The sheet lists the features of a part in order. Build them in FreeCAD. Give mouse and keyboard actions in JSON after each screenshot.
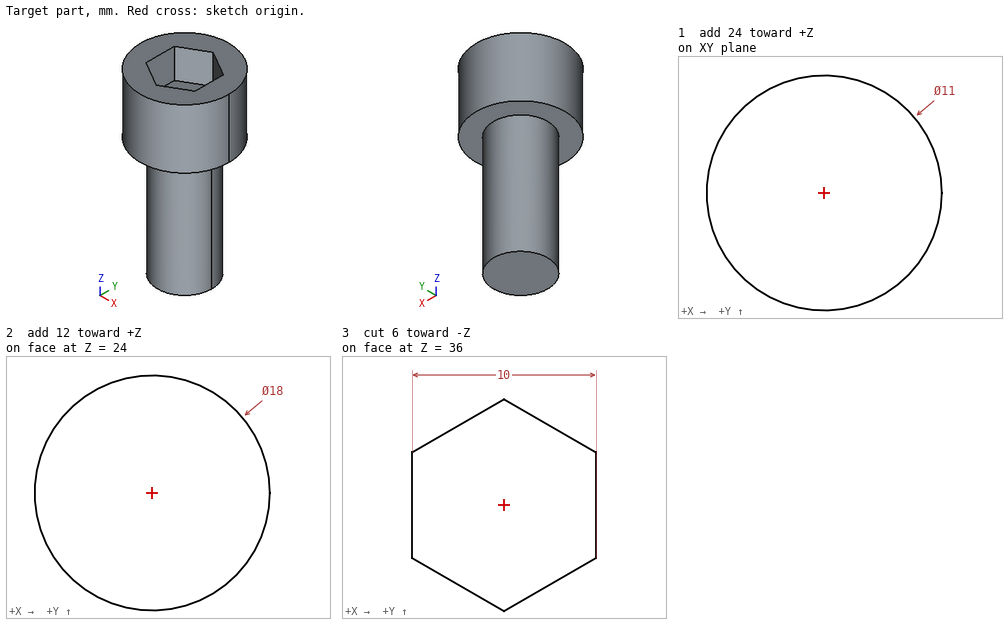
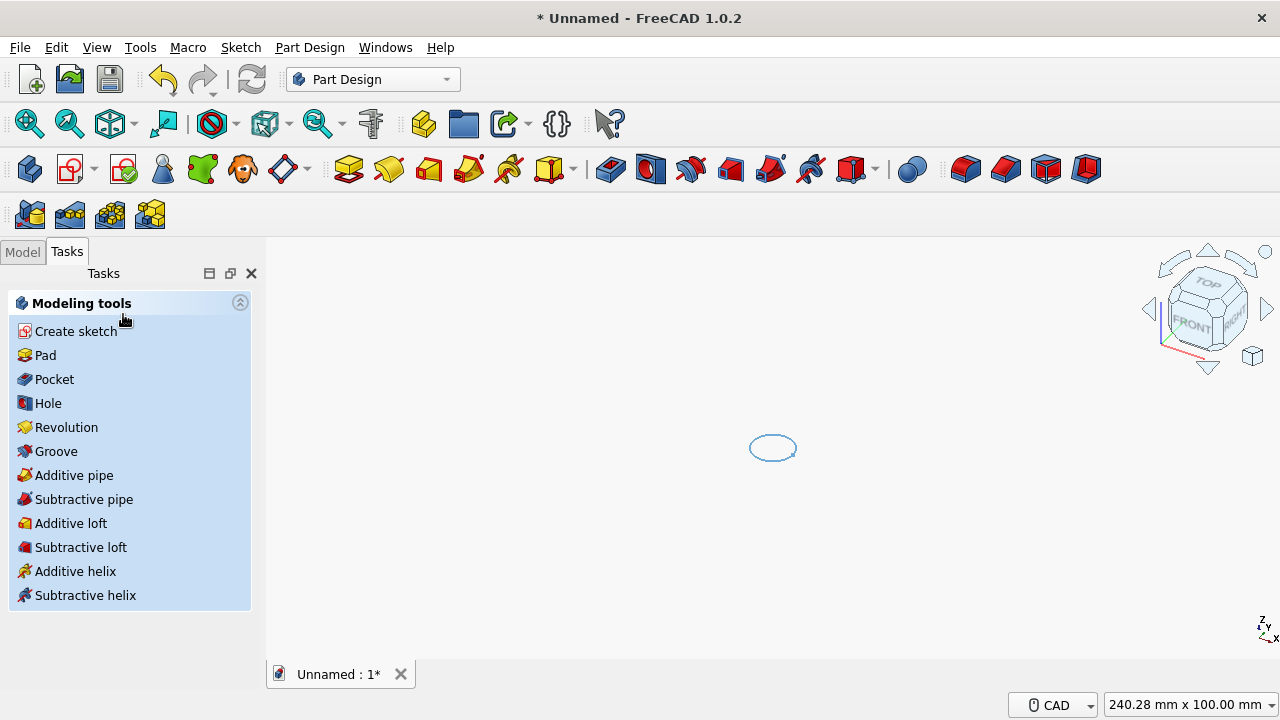
{"action": "left_click", "coordinate": [350, 170]}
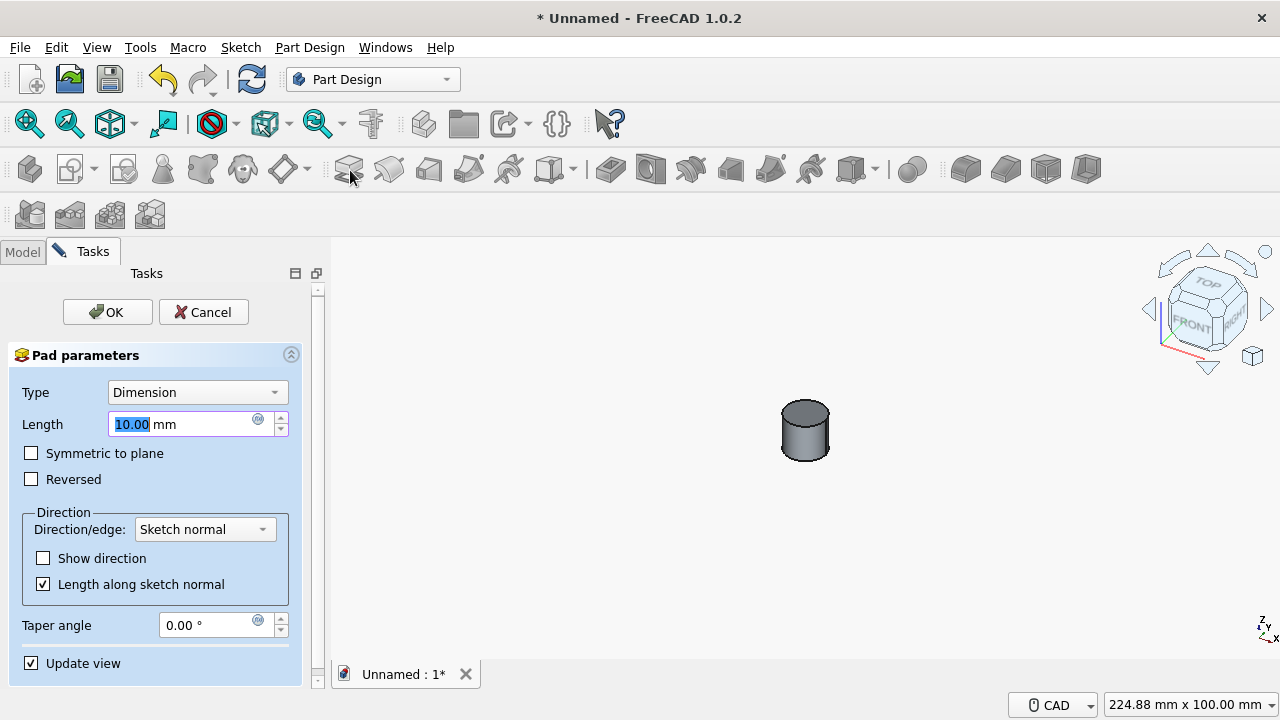
{"action": "type", "text": "24"}
{"action": "key", "text": "Tab"}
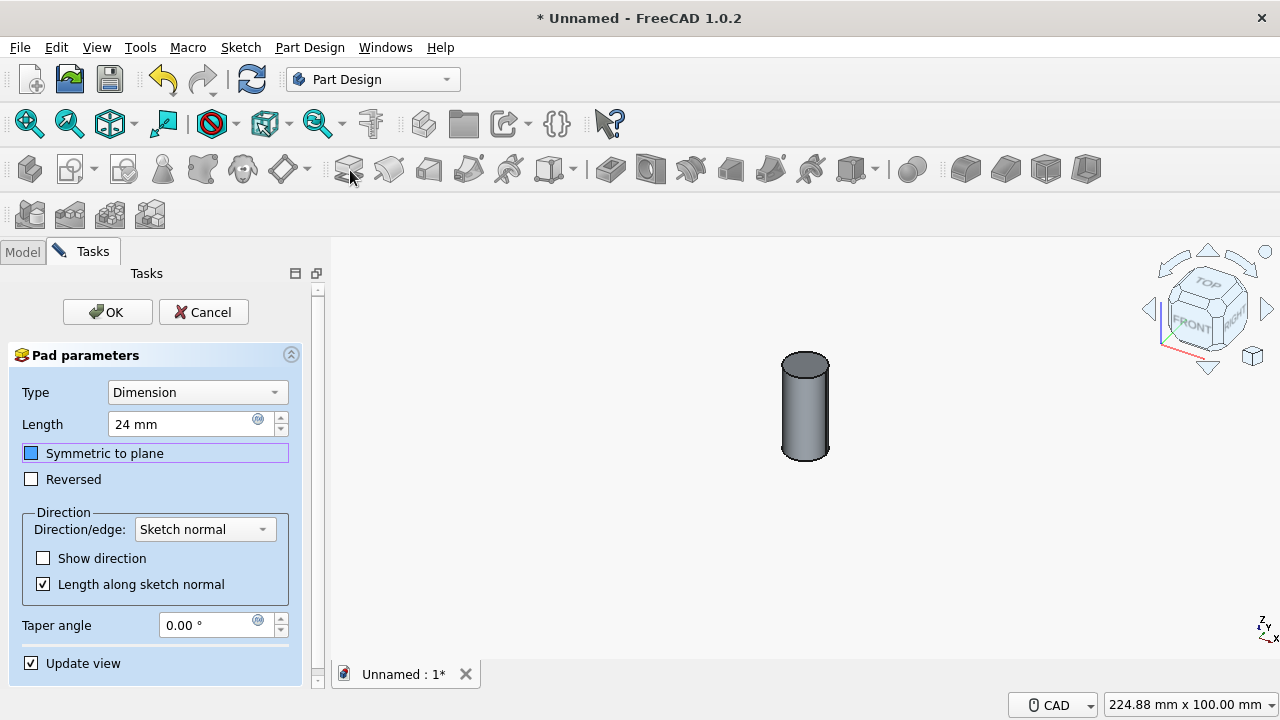
{"action": "left_click", "coordinate": [108, 312]}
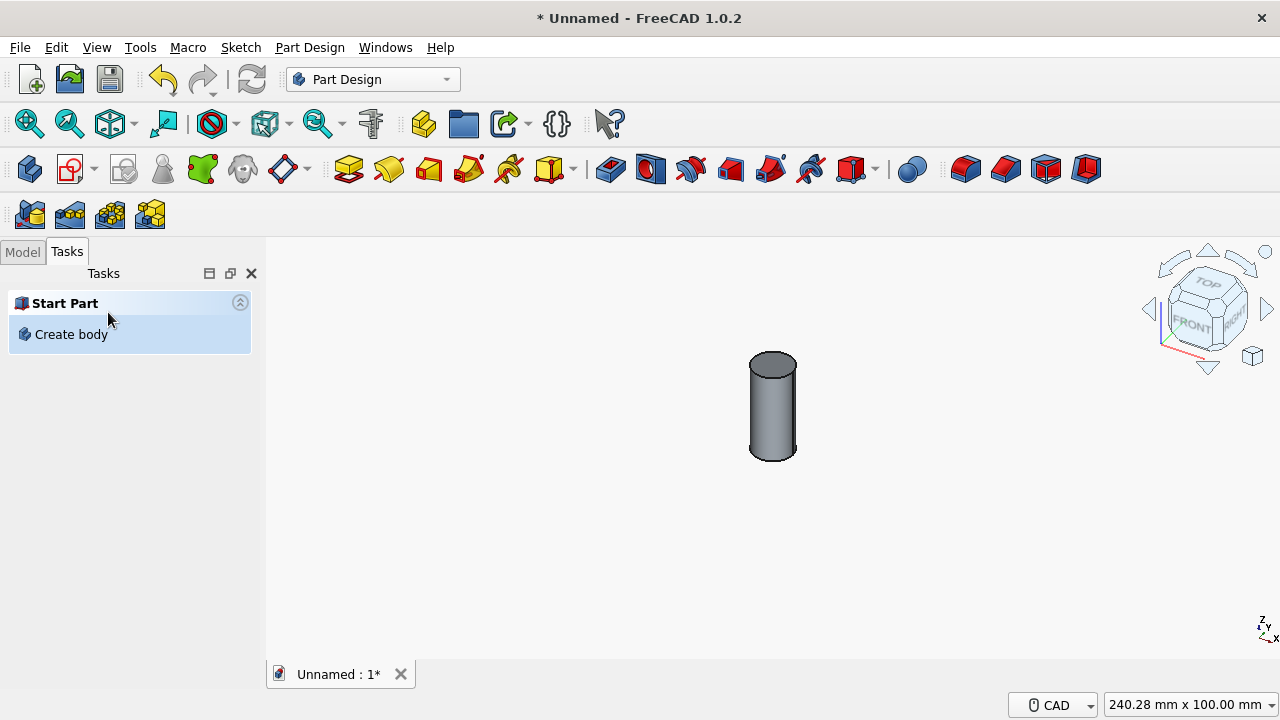
{"action": "left_click", "coordinate": [30, 124]}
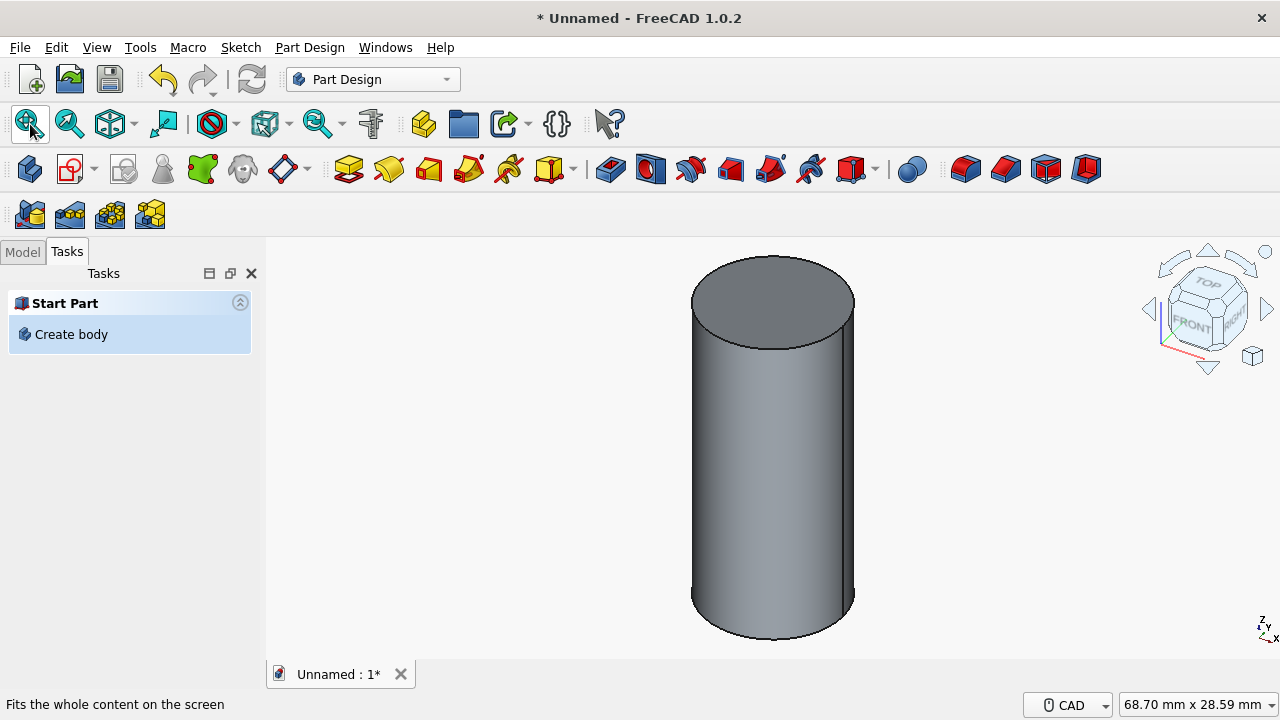
{"action": "left_click", "coordinate": [773, 302]}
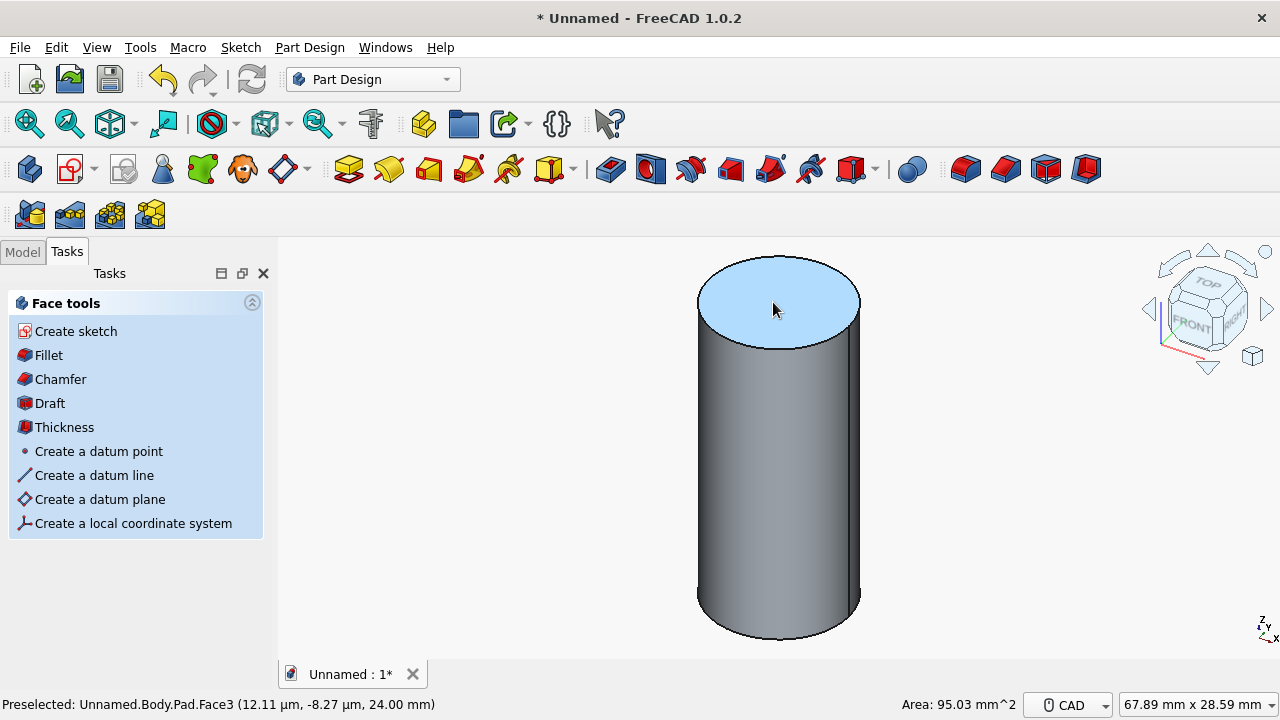
{"action": "left_click", "coordinate": [70, 170]}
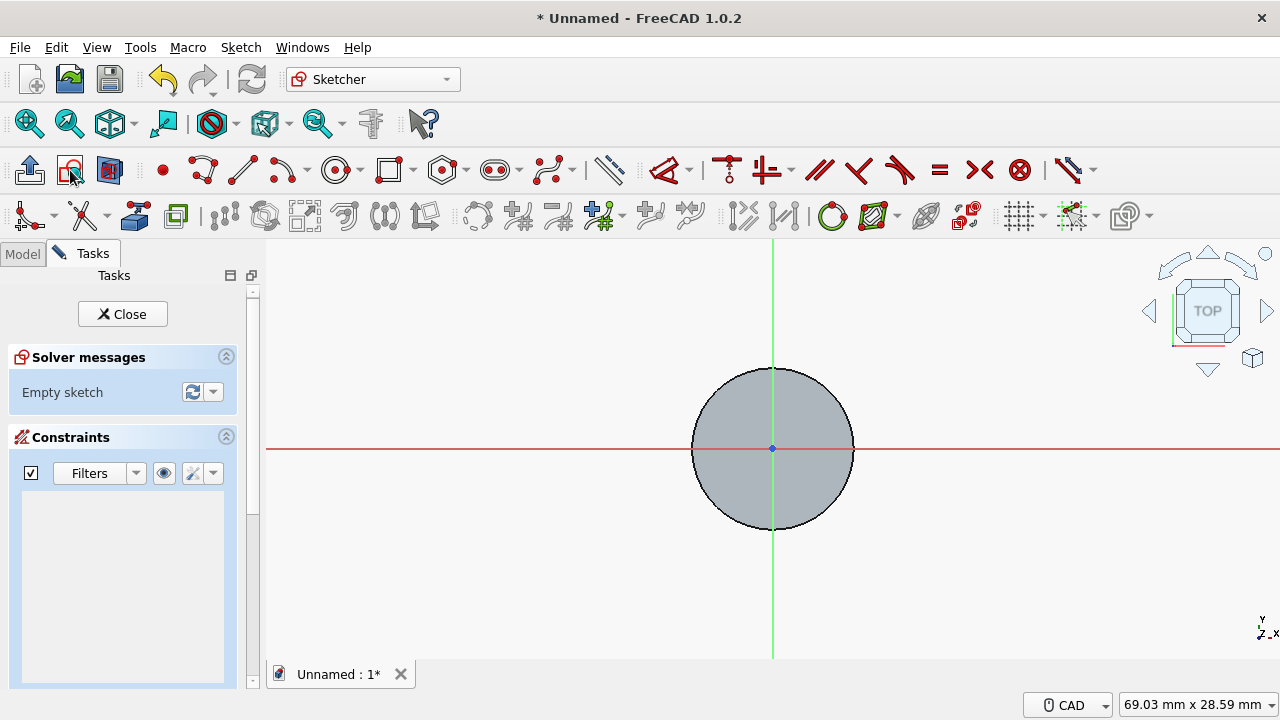
{"action": "left_click", "coordinate": [336, 170]}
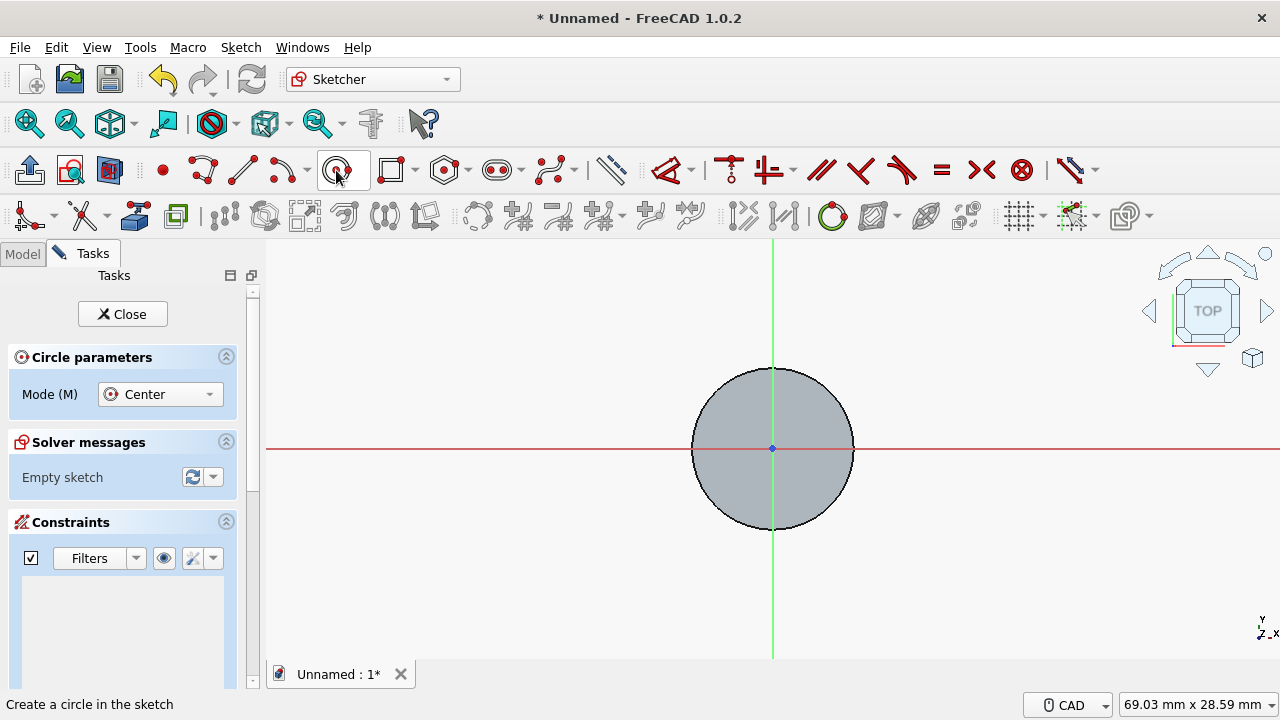
{"action": "left_click", "coordinate": [773, 449]}
{"action": "left_click", "coordinate": [866, 356]}
{"action": "key", "text": "Escape"}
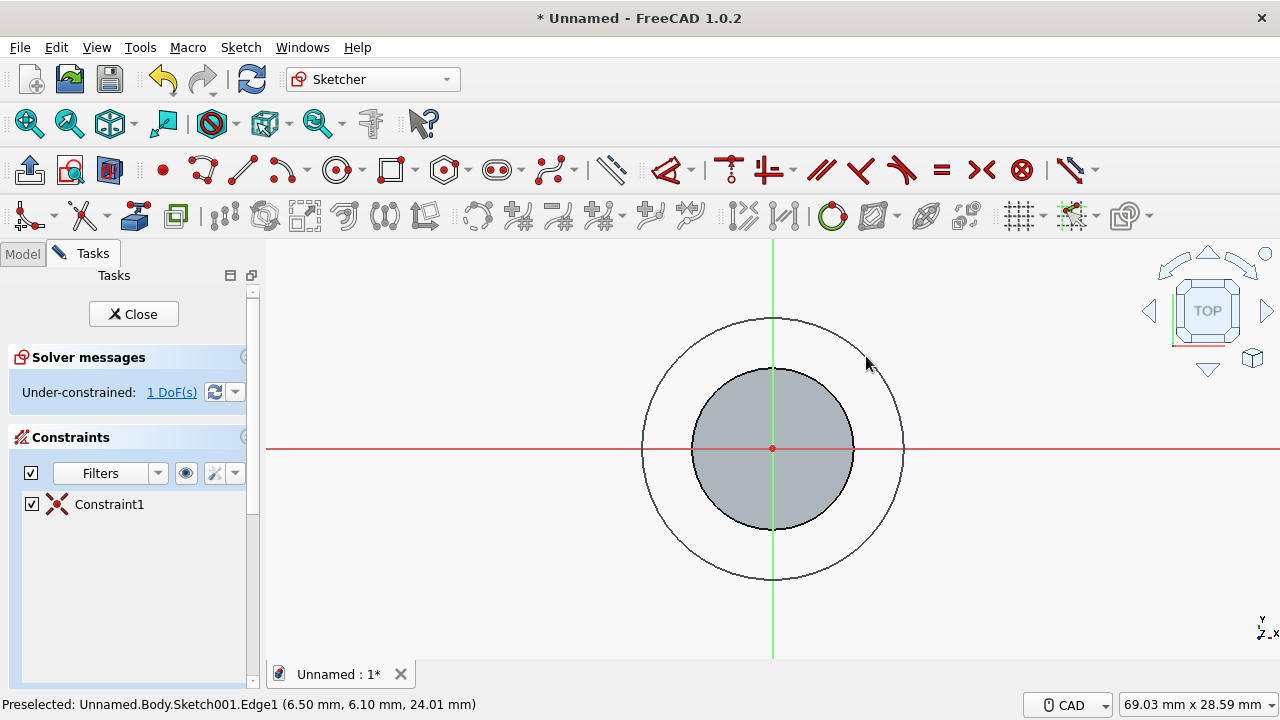
{"action": "left_click", "coordinate": [666, 170]}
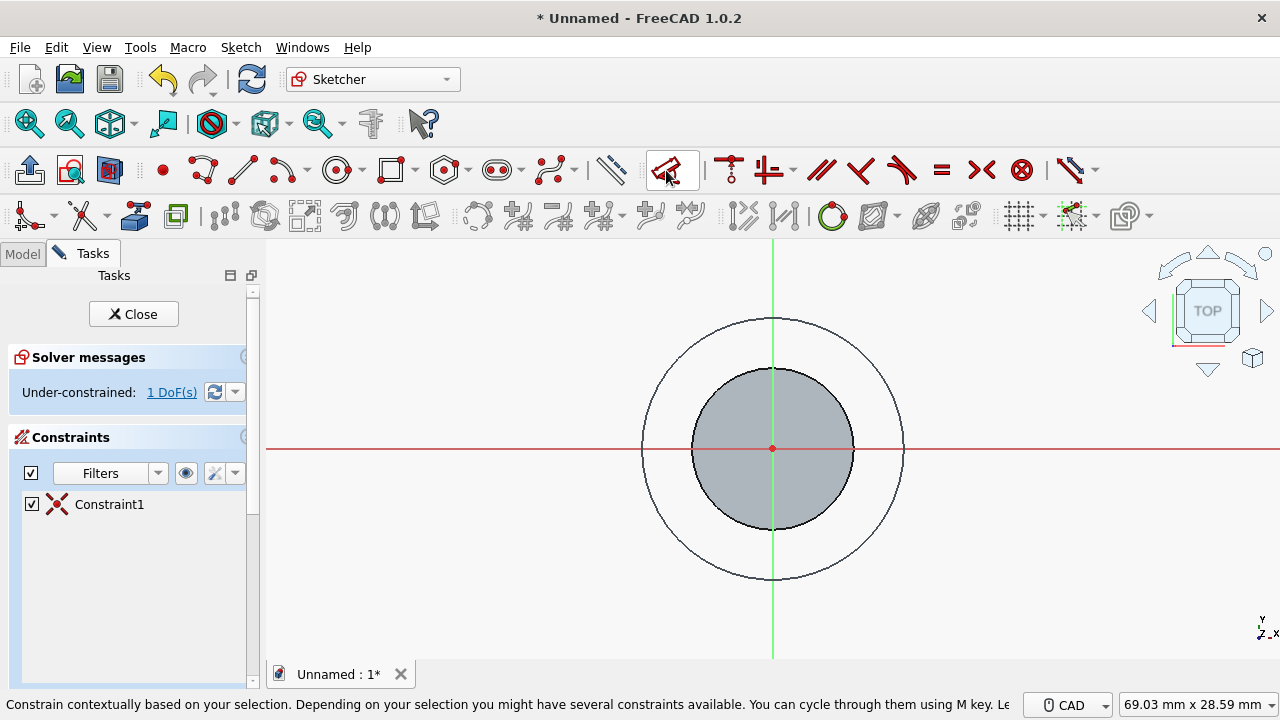
{"action": "left_click", "coordinate": [865, 356]}
{"action": "left_click", "coordinate": [888, 333]}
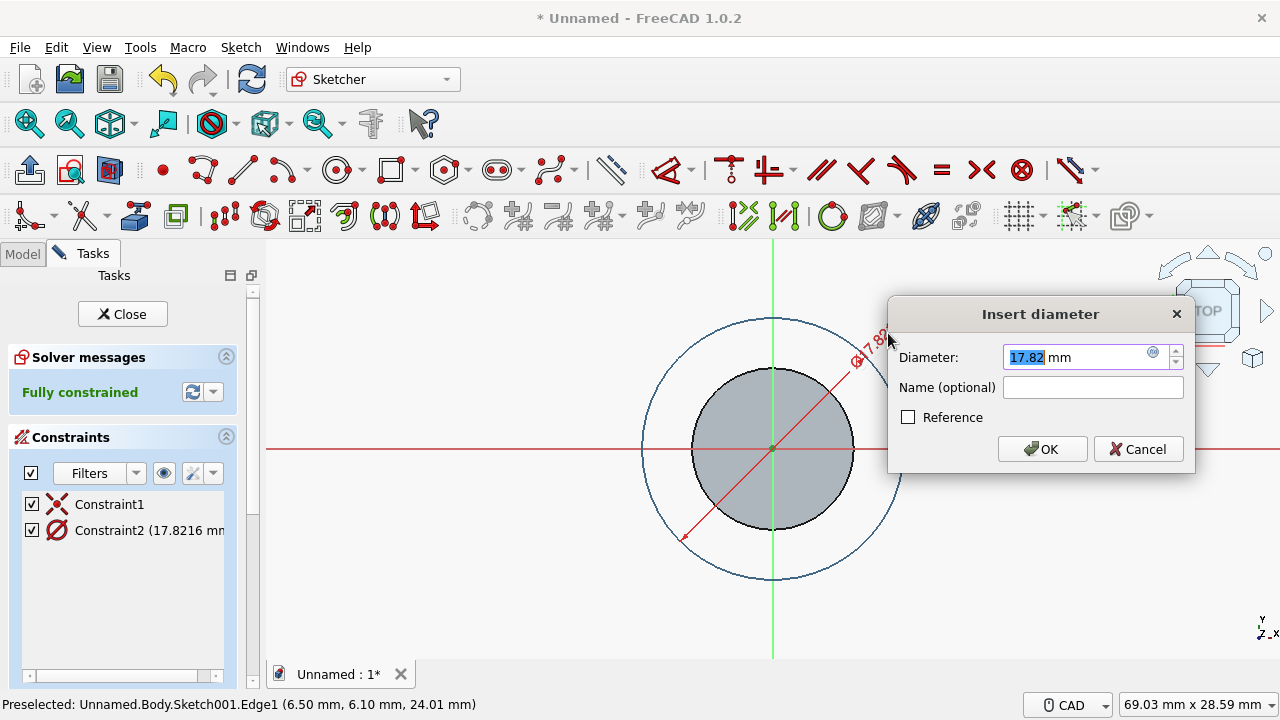
{"action": "type", "text": "18"}
{"action": "key", "text": "Return"}
{"action": "key", "text": "Escape"}